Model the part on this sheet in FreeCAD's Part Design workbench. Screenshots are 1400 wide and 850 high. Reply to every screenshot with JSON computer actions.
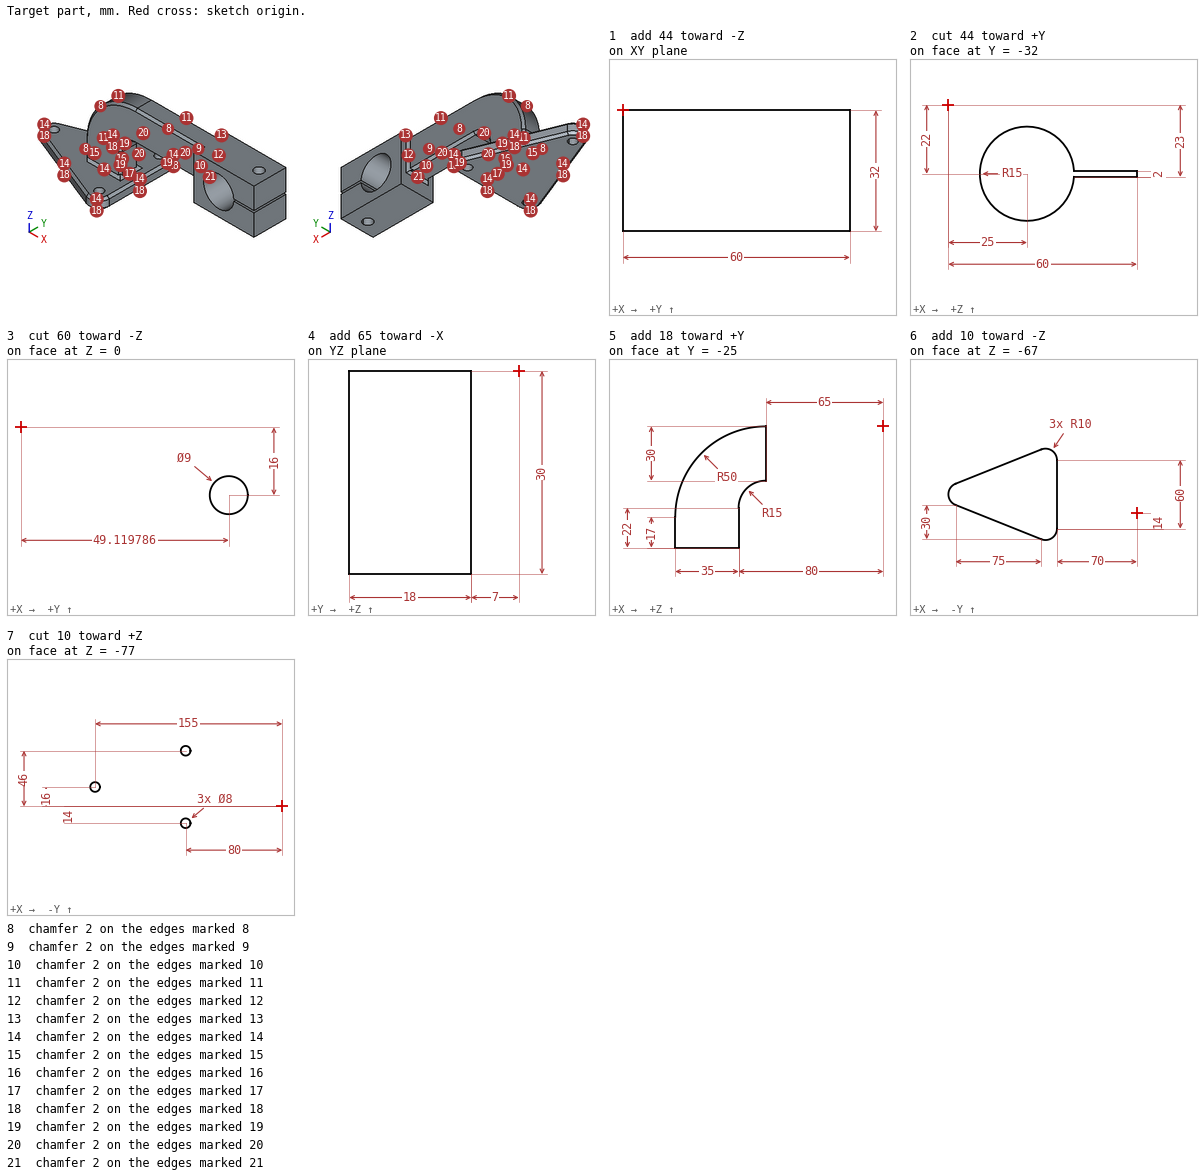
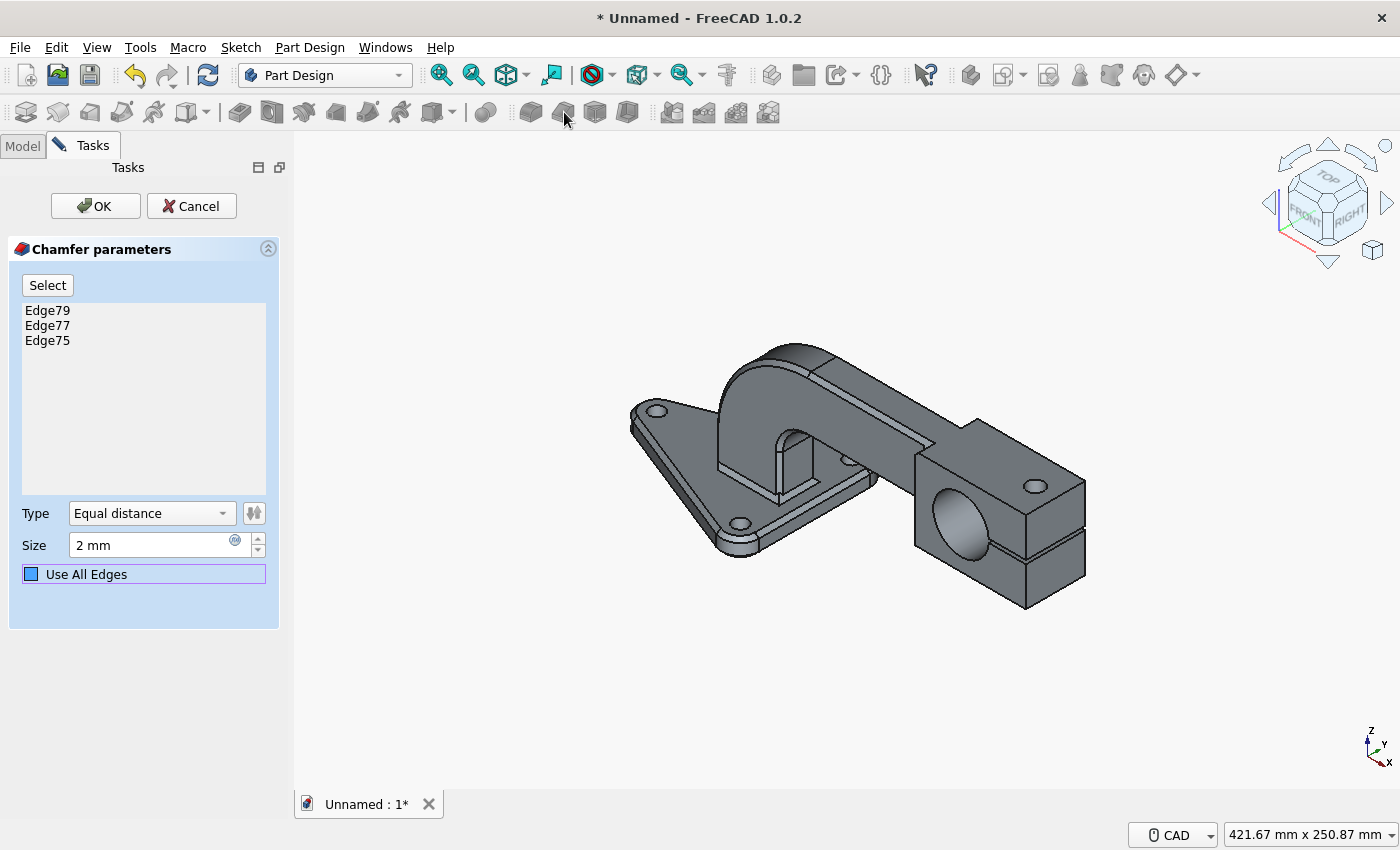
{"action": "left_click", "coordinate": [96, 206]}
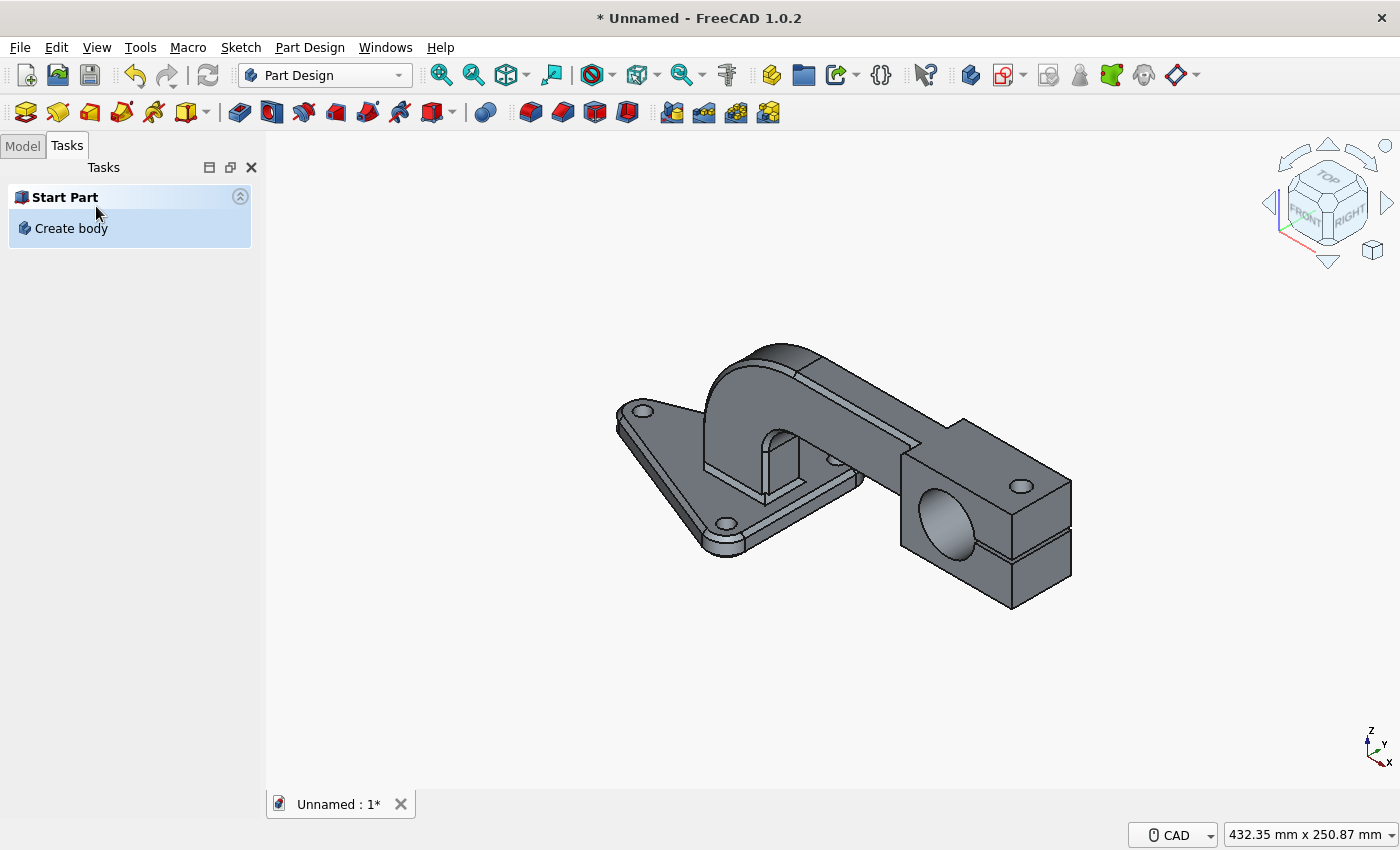
{"action": "key", "text": "2"}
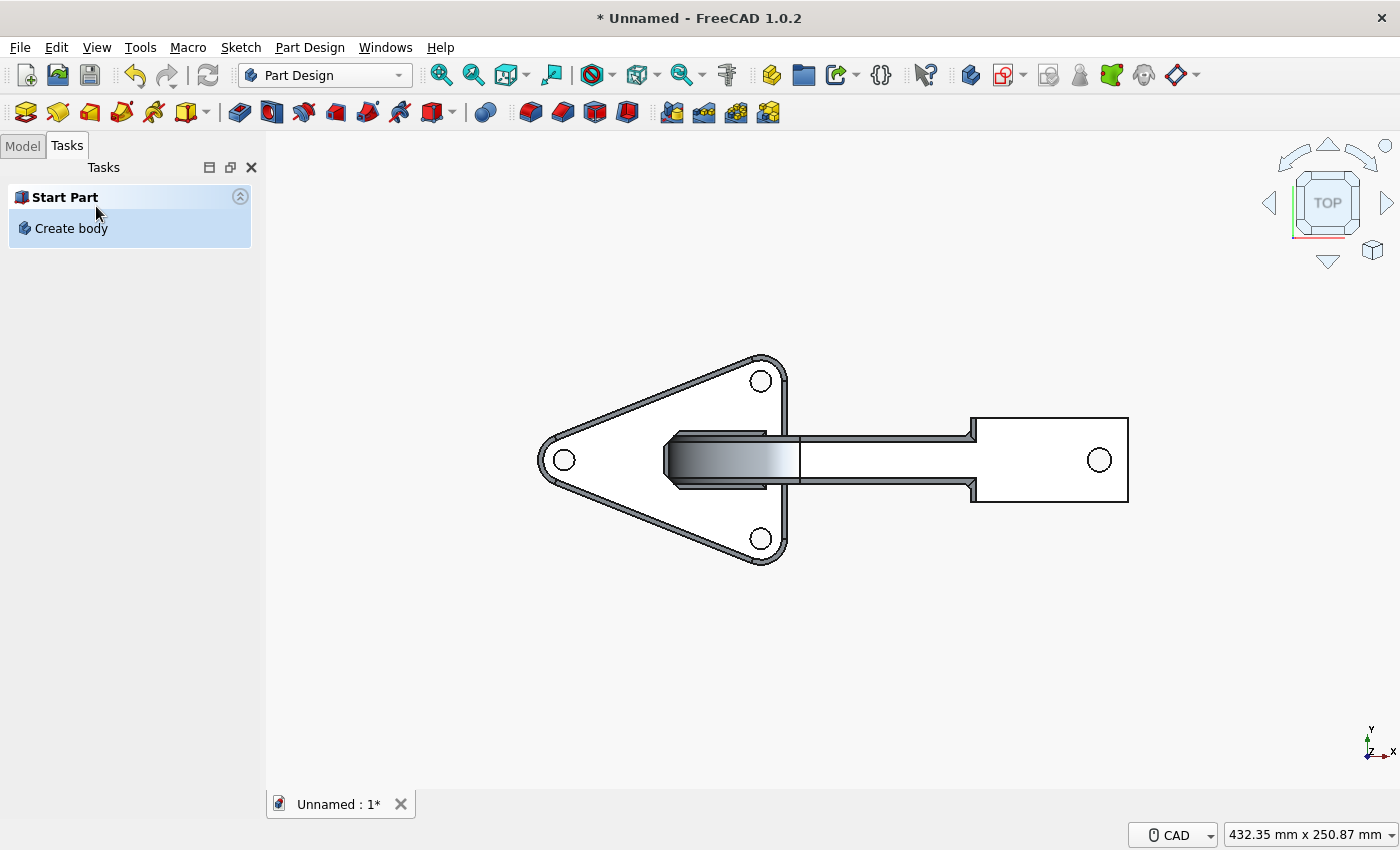
{"action": "key", "text": "0"}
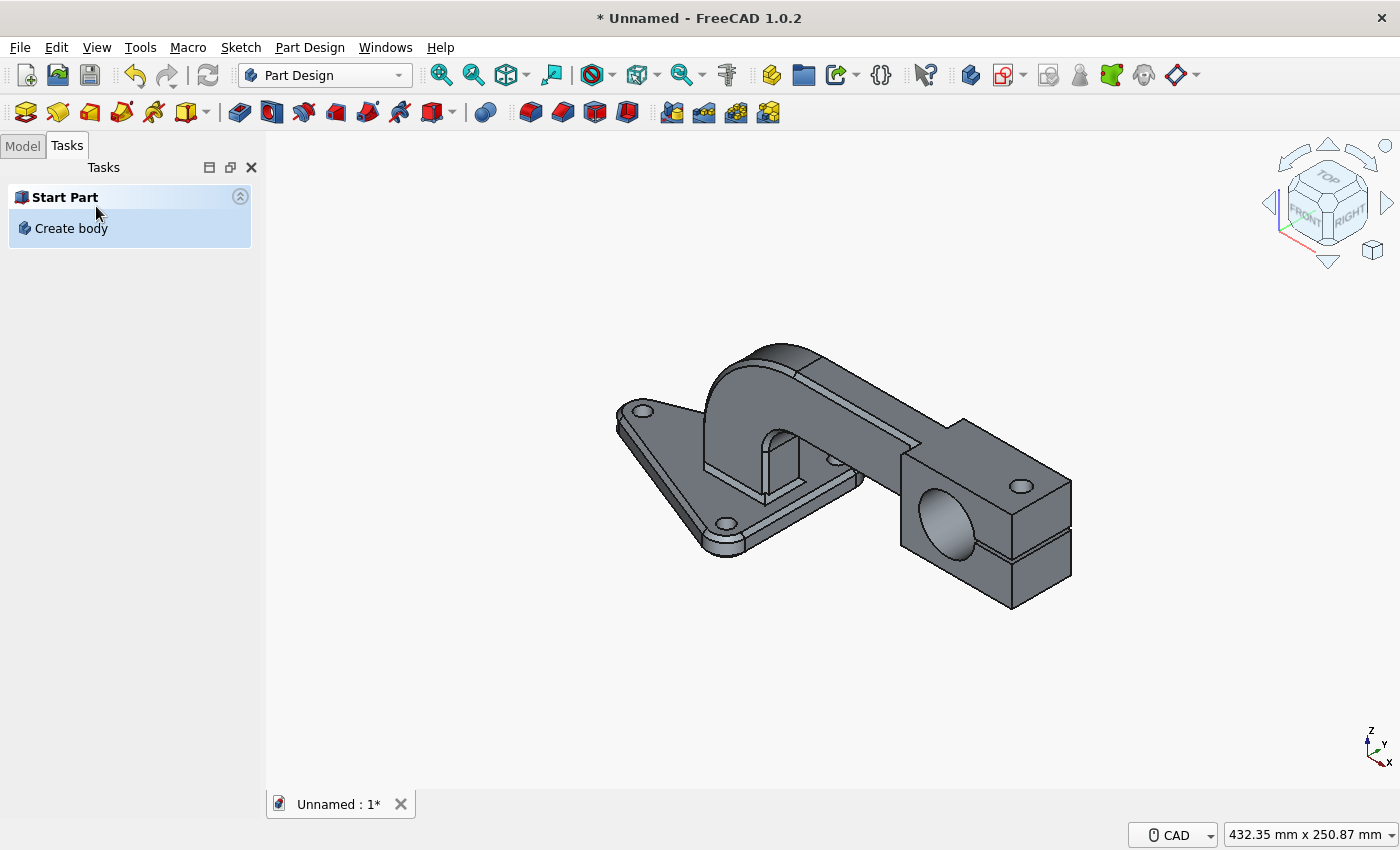
{"action": "key", "text": "1"}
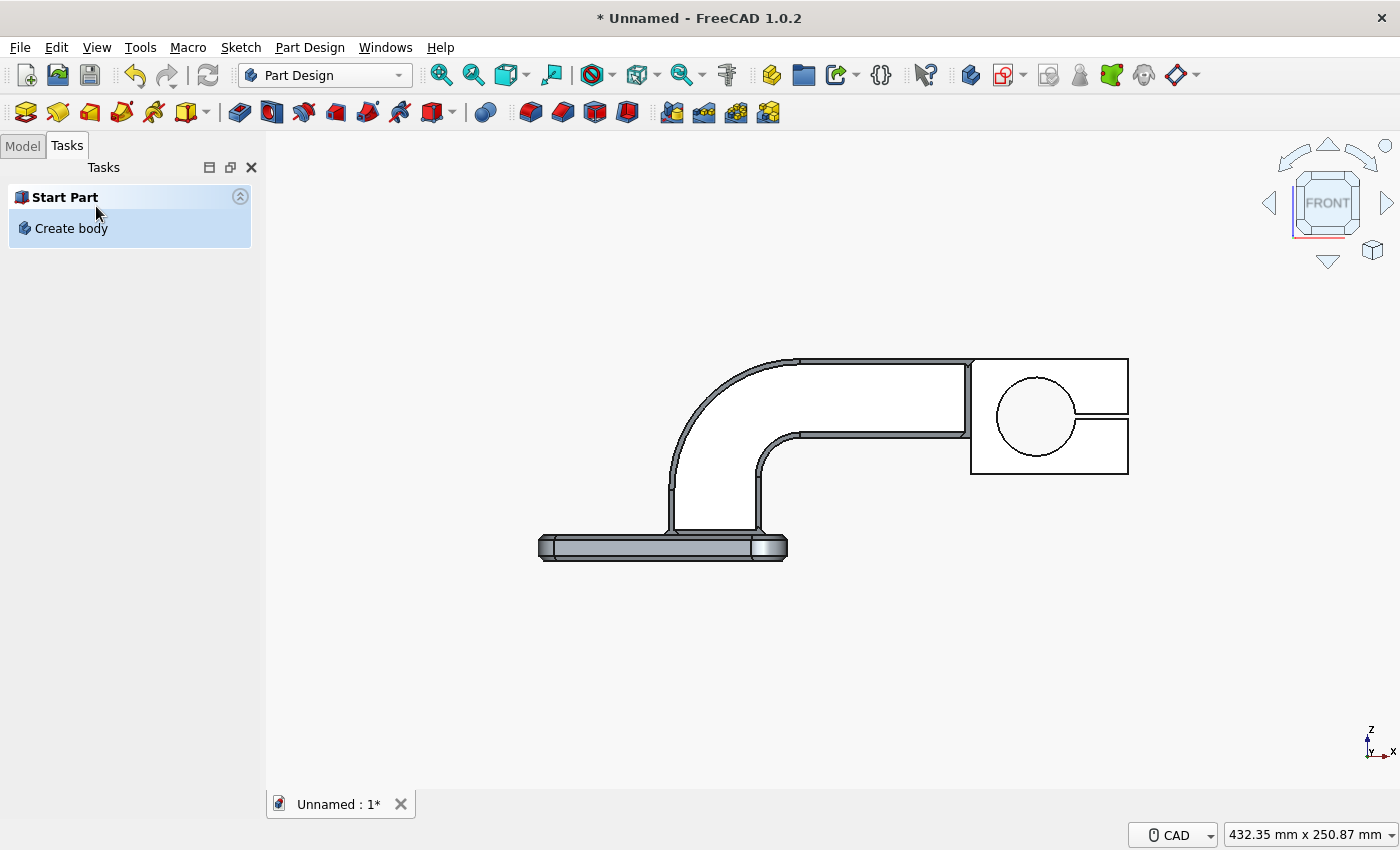
{"action": "key", "text": "3"}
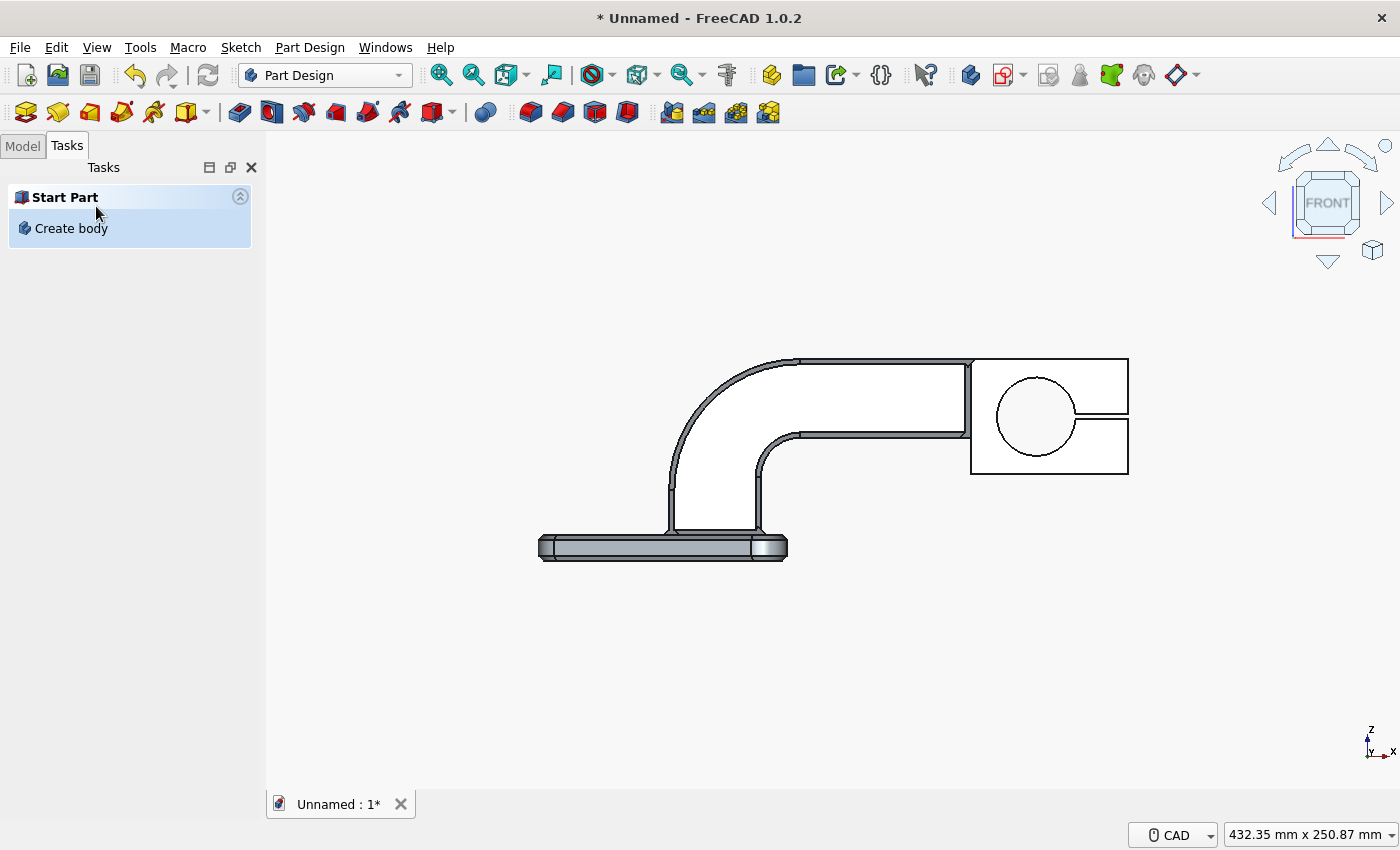
{"action": "left_click", "coordinate": [442, 76]}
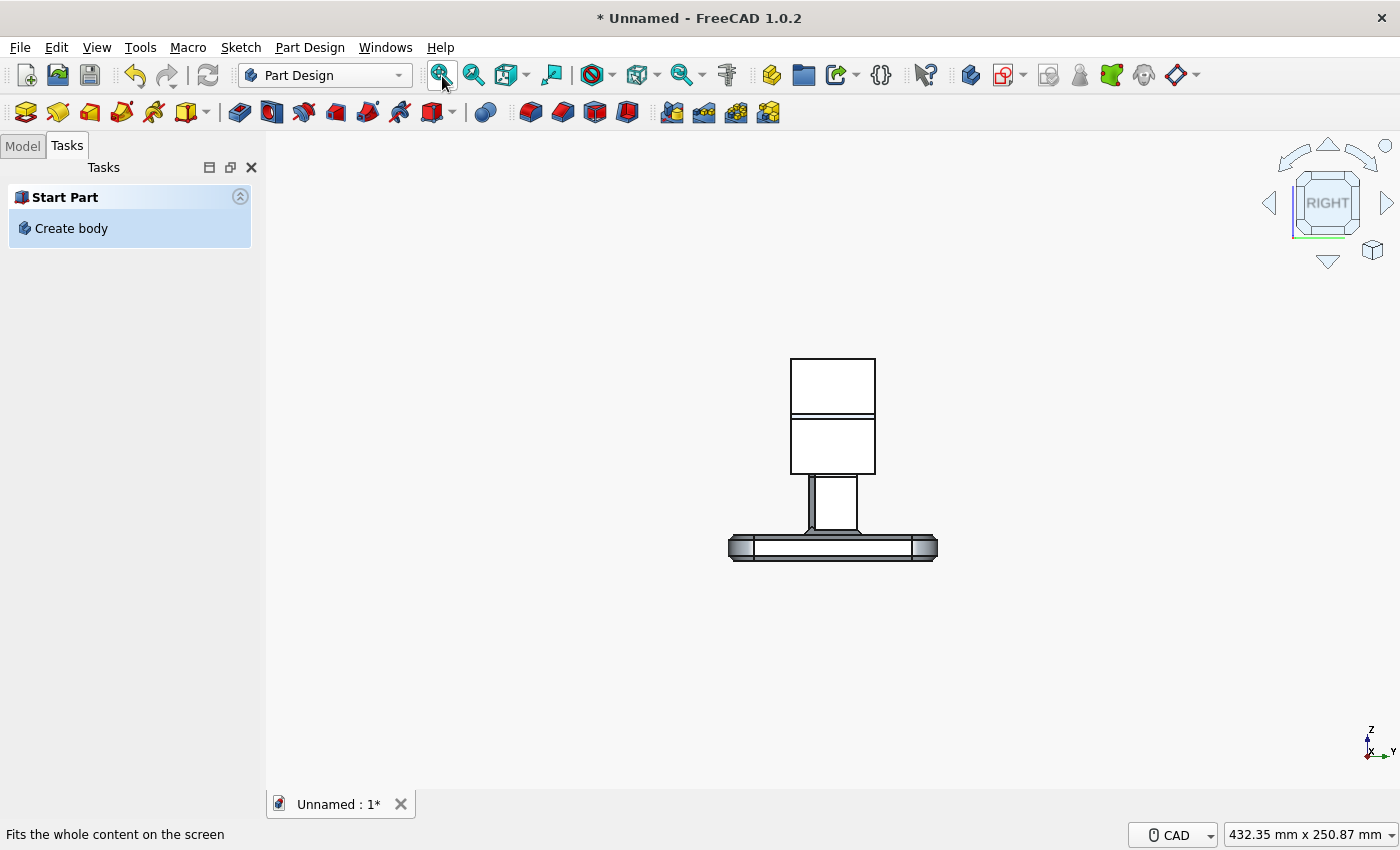
{"action": "left_click", "coordinate": [857, 502]}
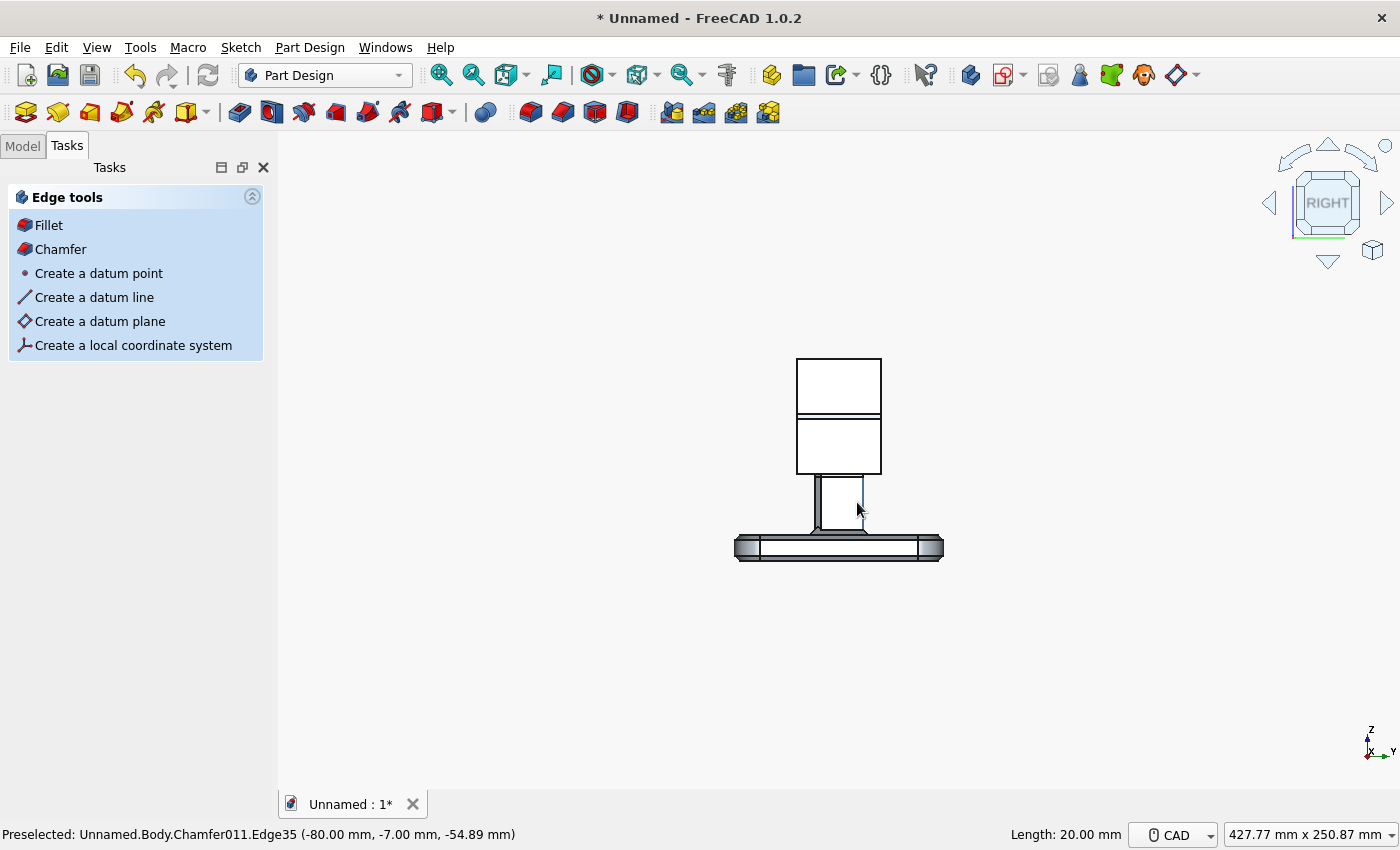
{"action": "key", "text": "5"}